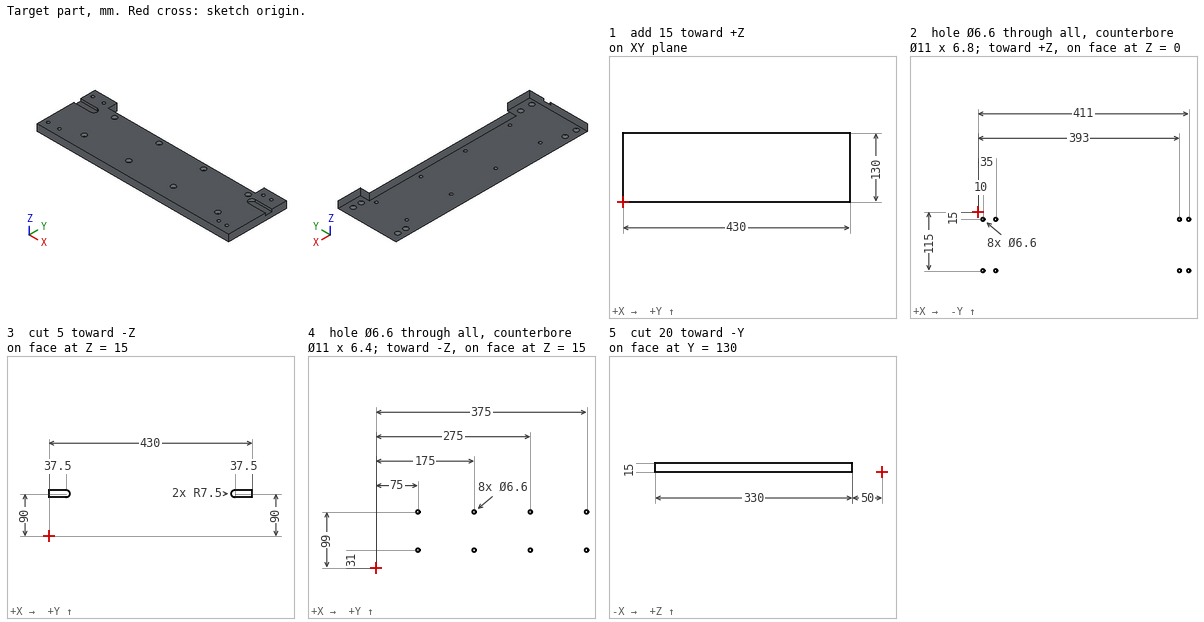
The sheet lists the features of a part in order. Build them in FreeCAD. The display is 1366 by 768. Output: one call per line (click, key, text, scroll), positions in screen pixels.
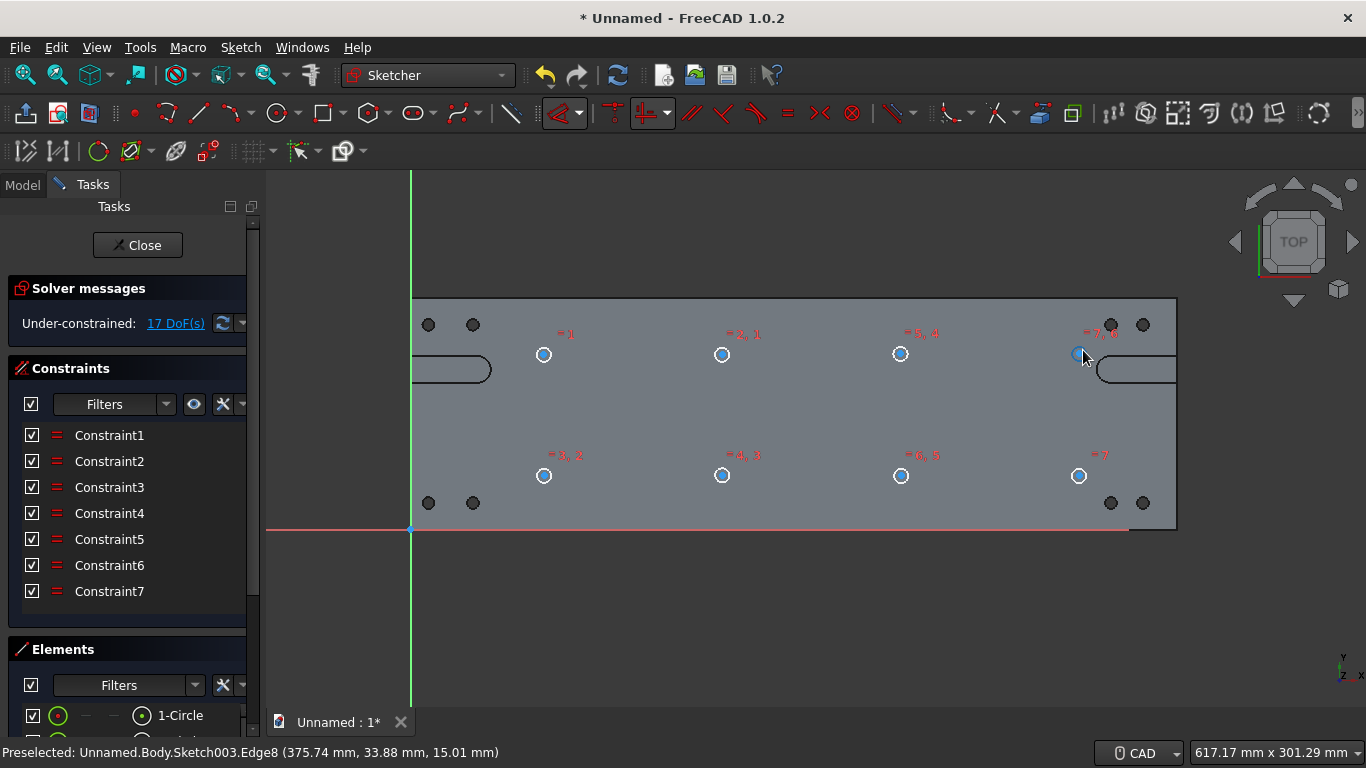
click(544, 355)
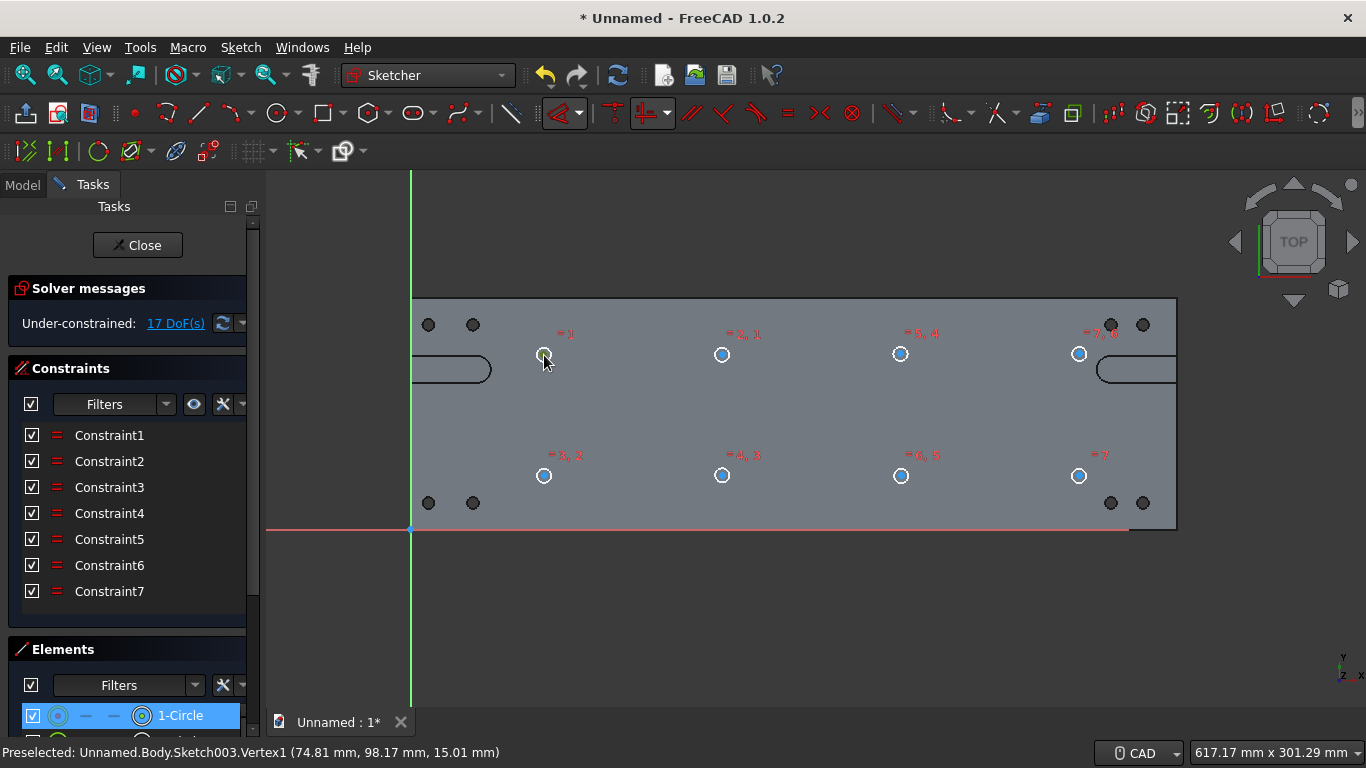
click(722, 355)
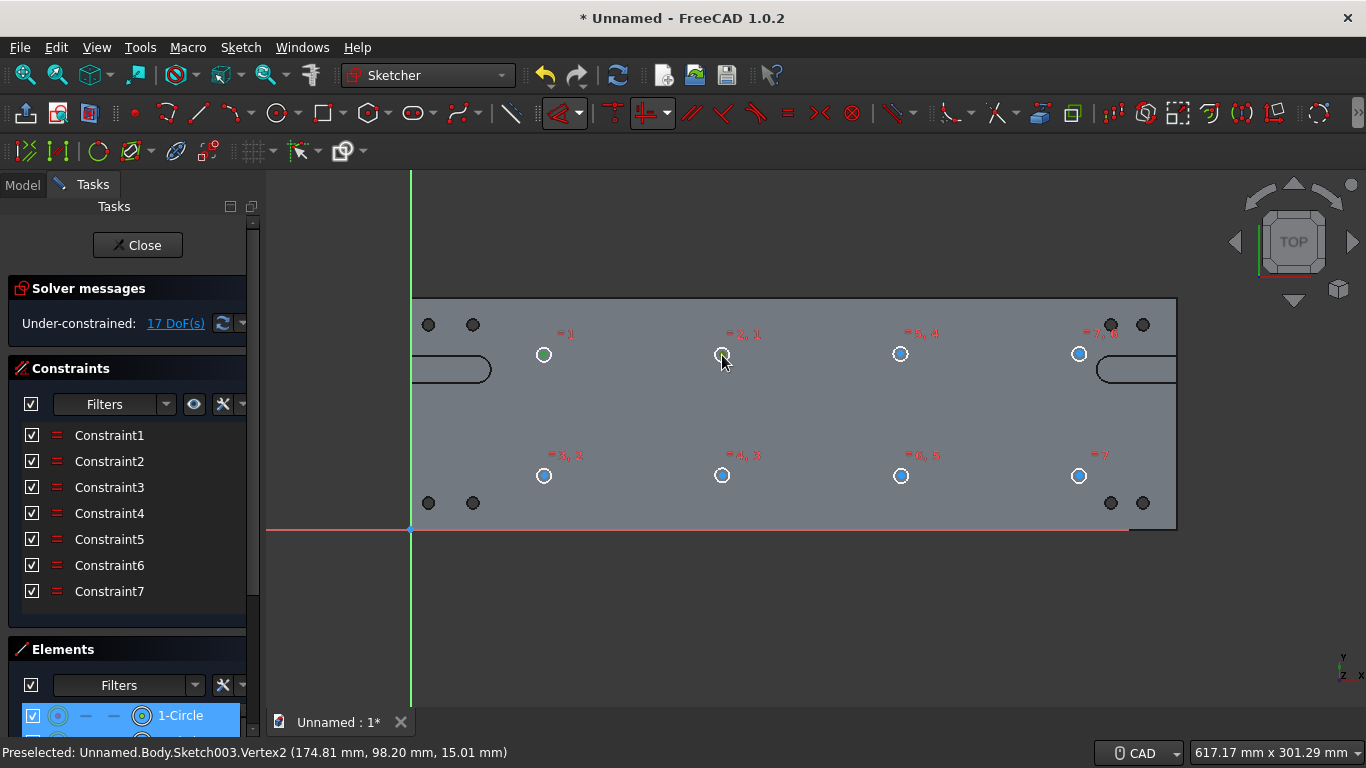
key(h)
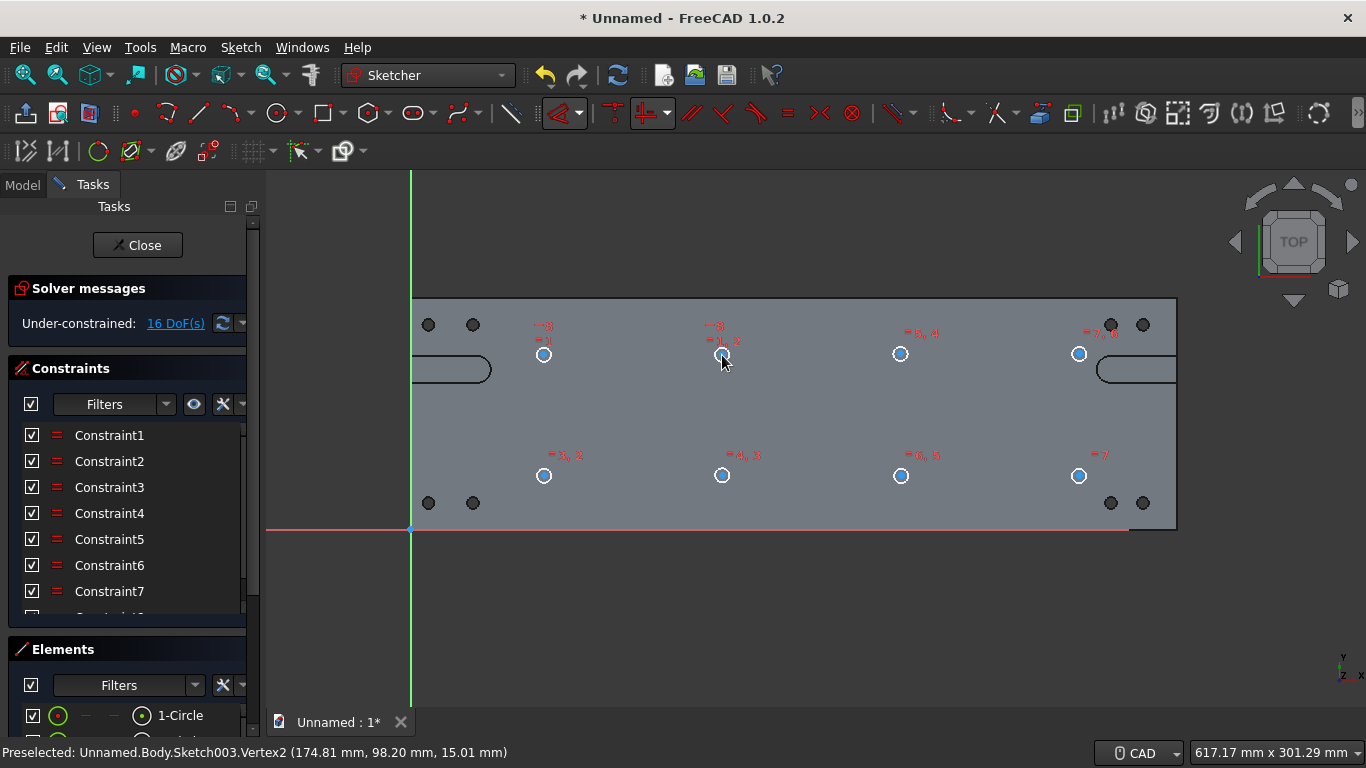
click(544, 355)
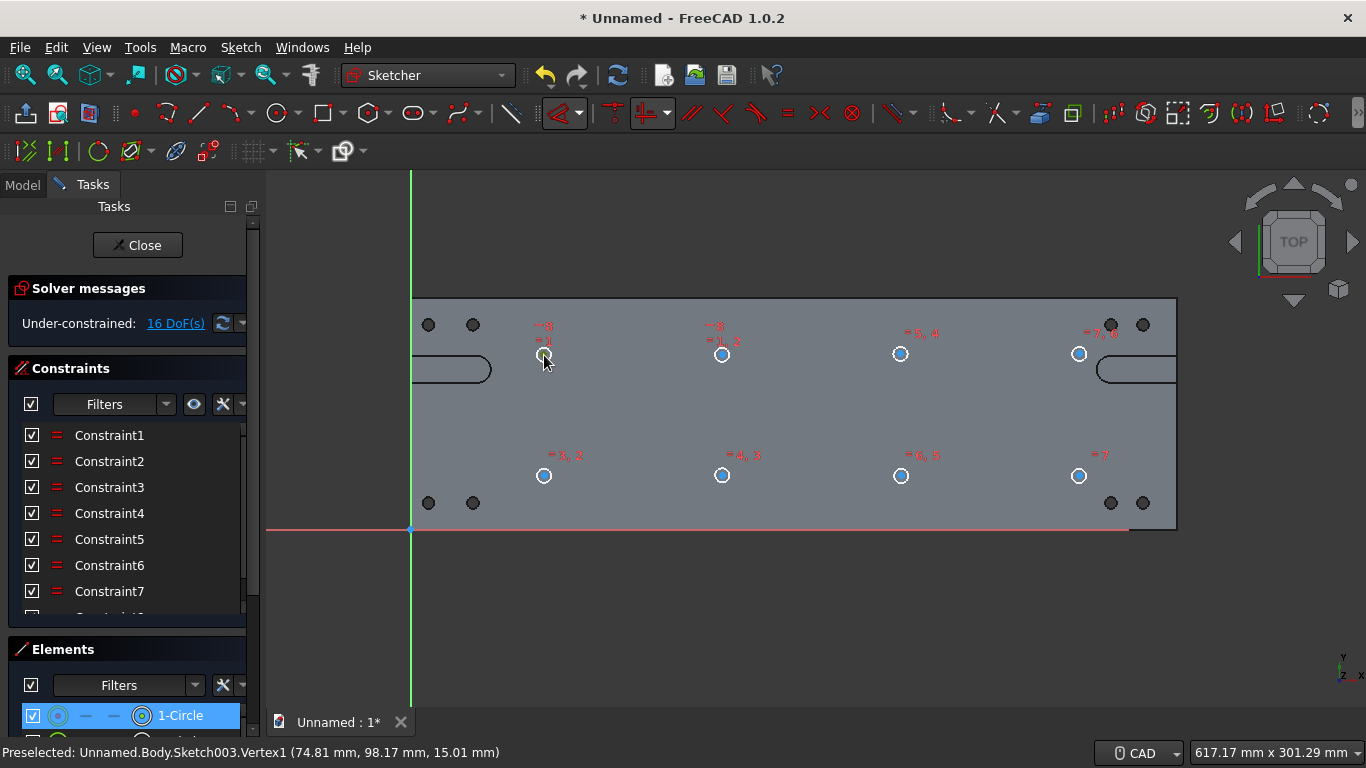
click(544, 476)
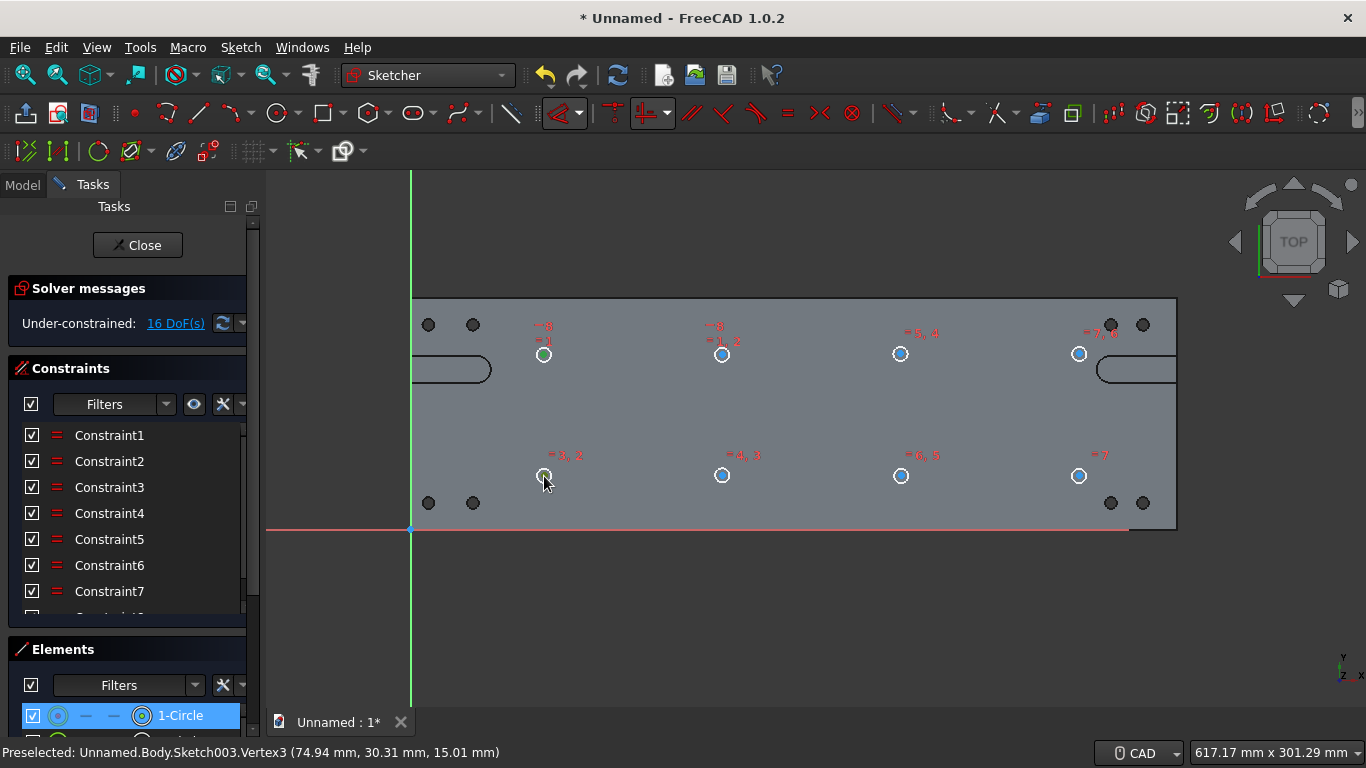
key(v)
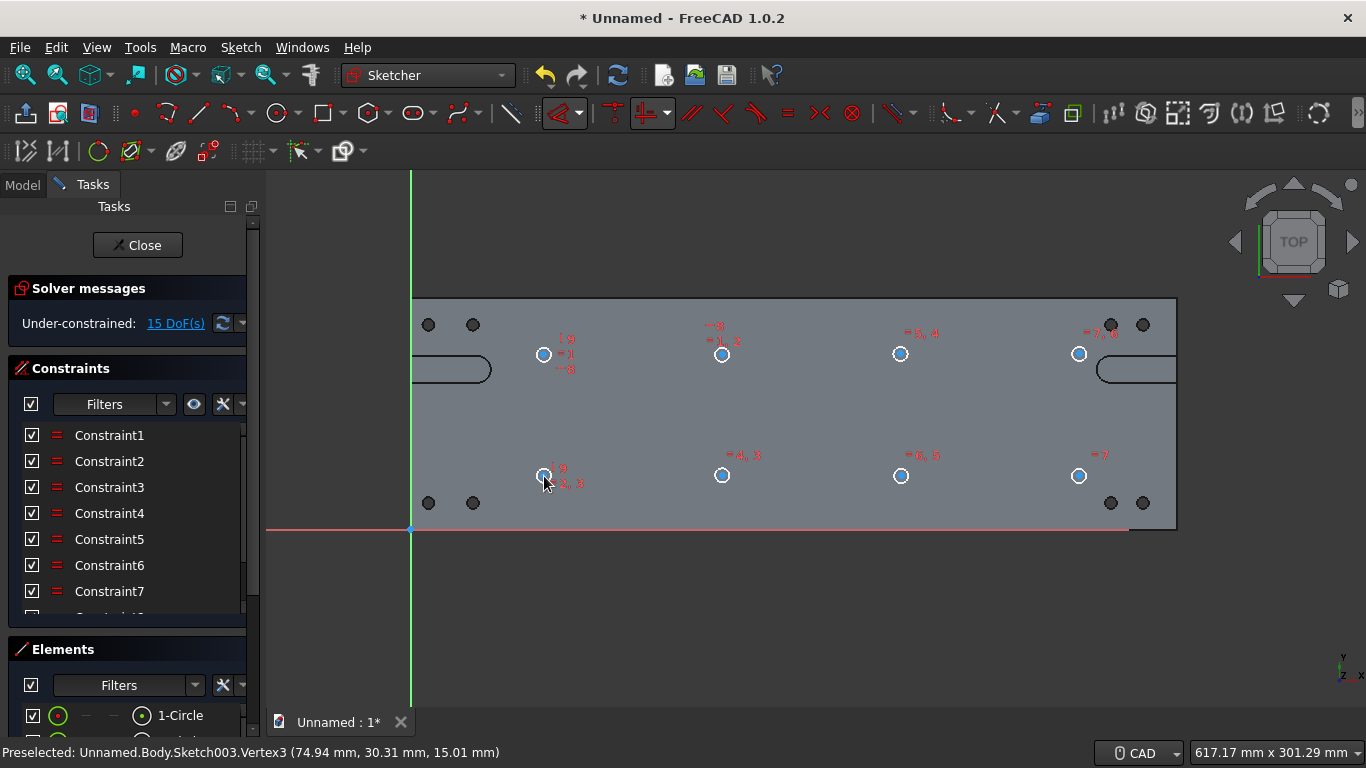
click(722, 355)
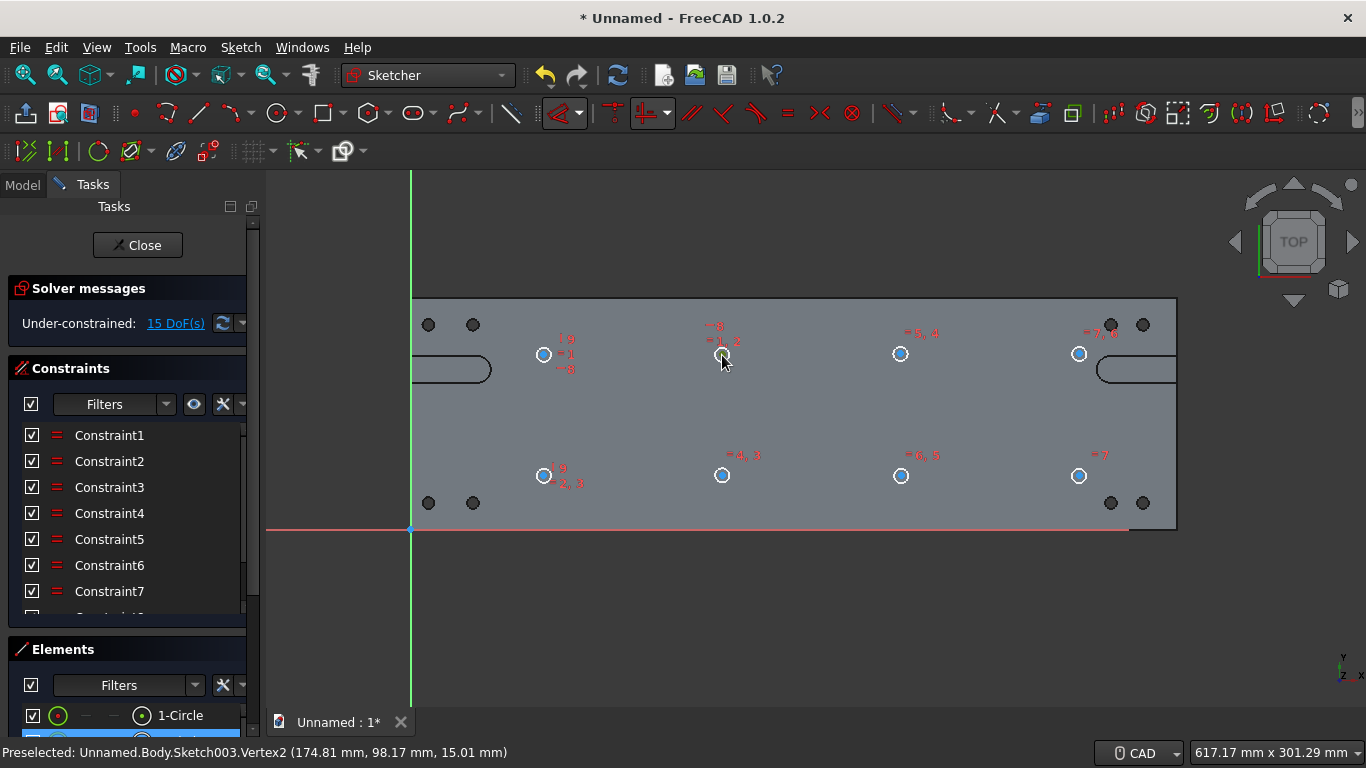
click(722, 475)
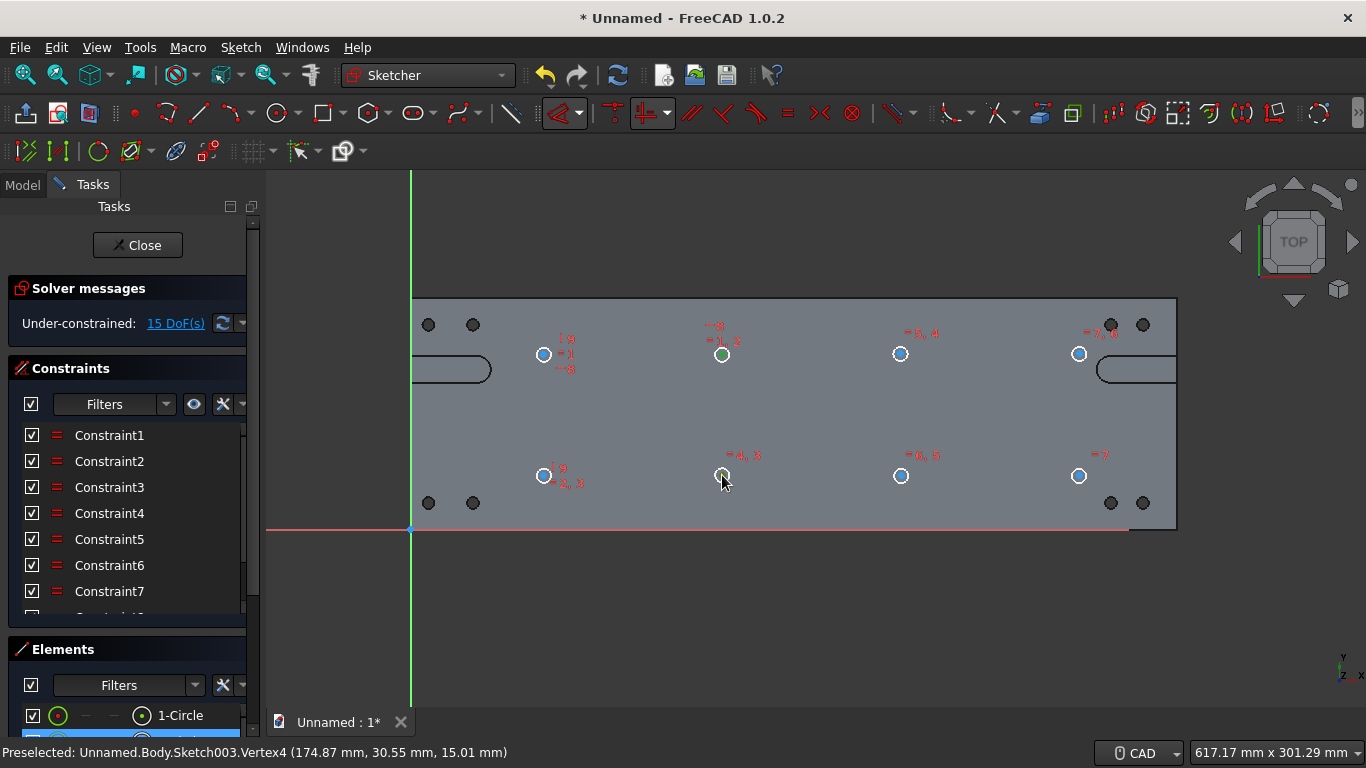
key(v)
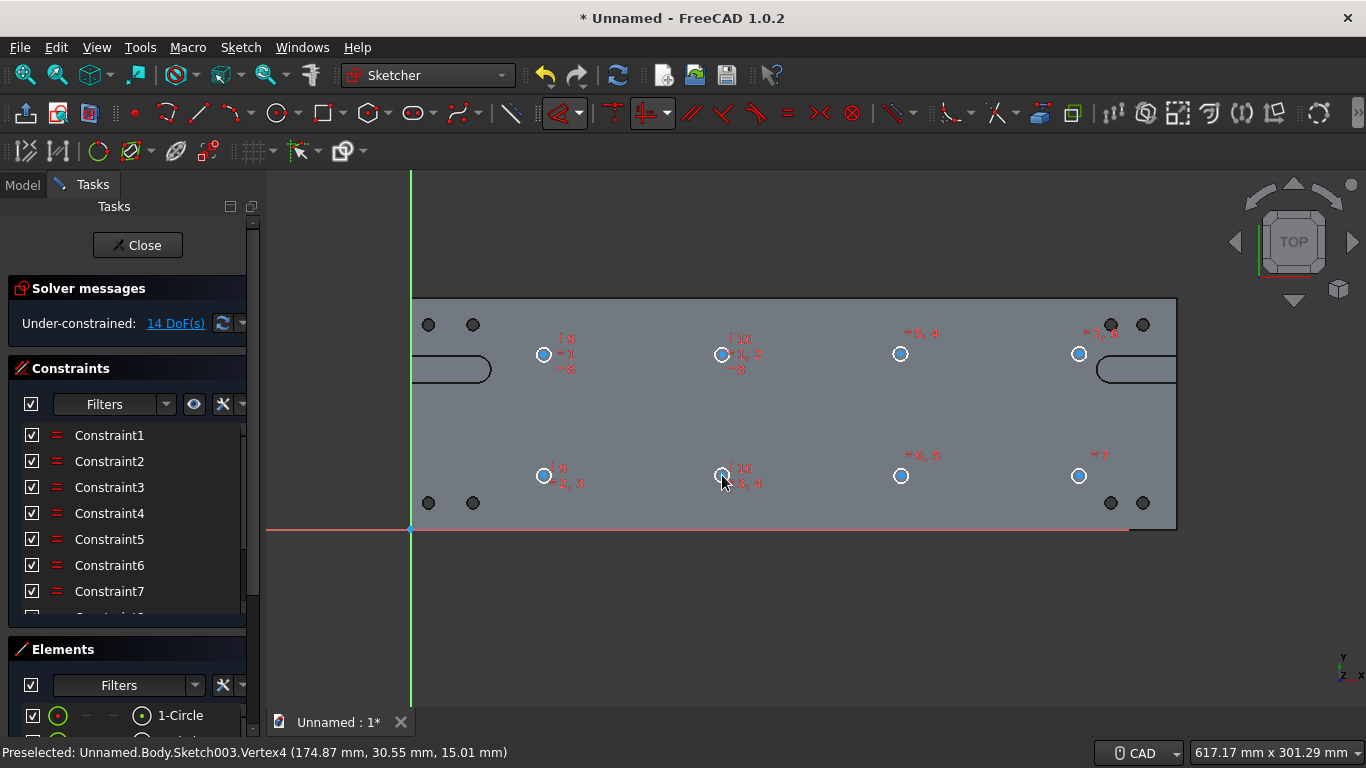
click(544, 476)